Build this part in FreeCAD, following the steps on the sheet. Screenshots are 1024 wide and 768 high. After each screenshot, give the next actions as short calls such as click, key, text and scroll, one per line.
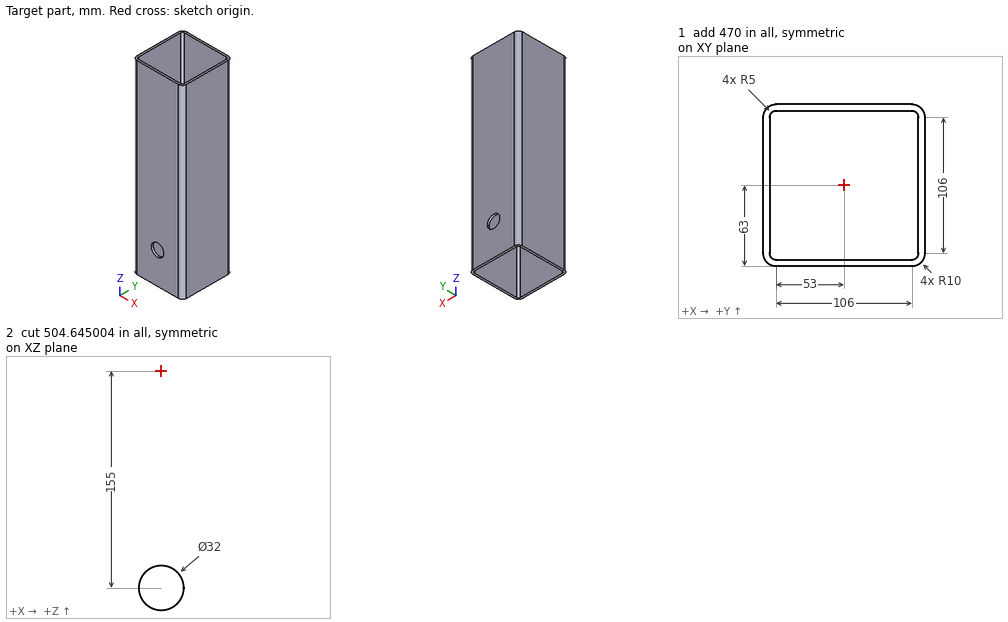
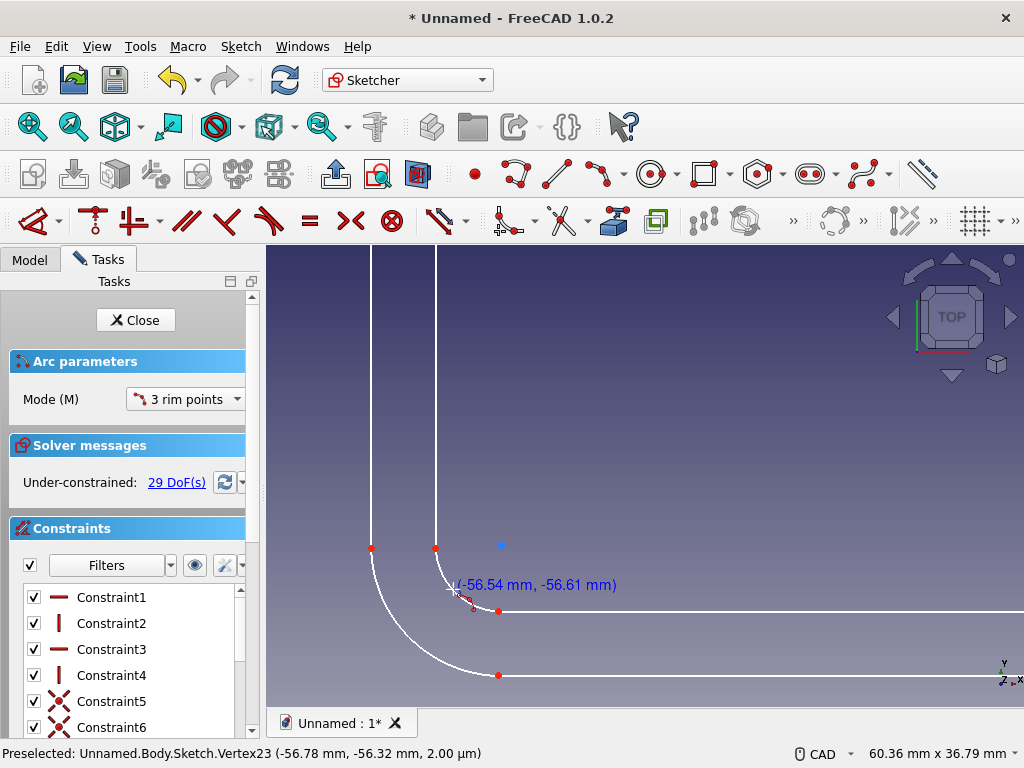
scroll(460, 594, down, 9)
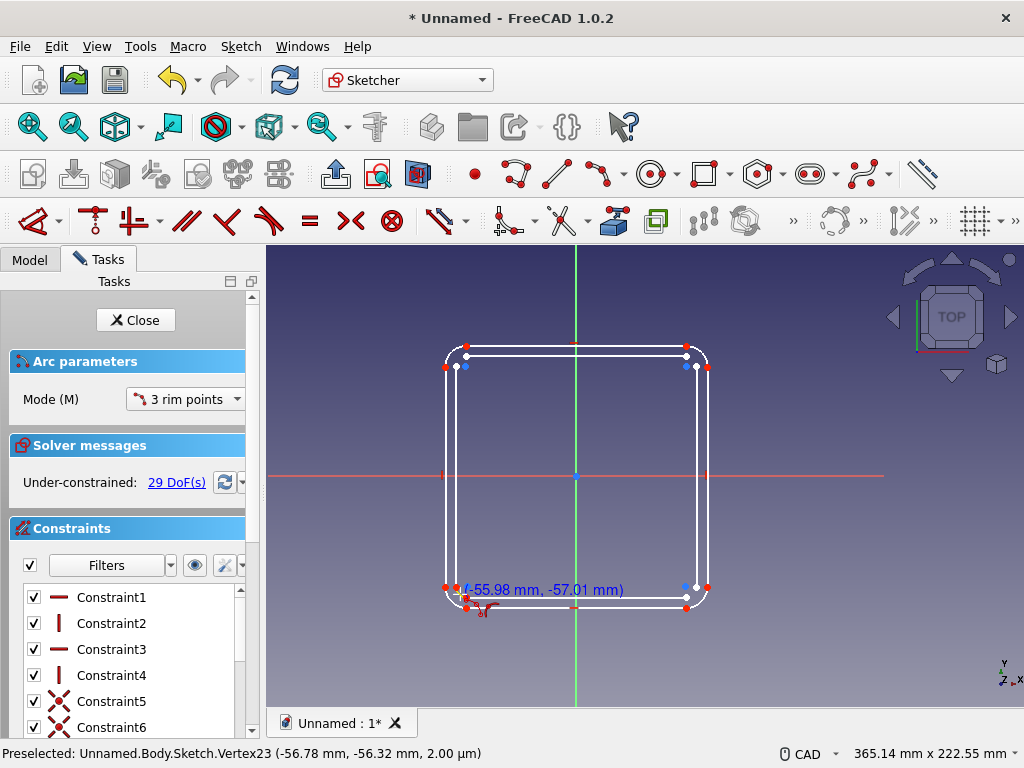
scroll(456, 366, up, 3)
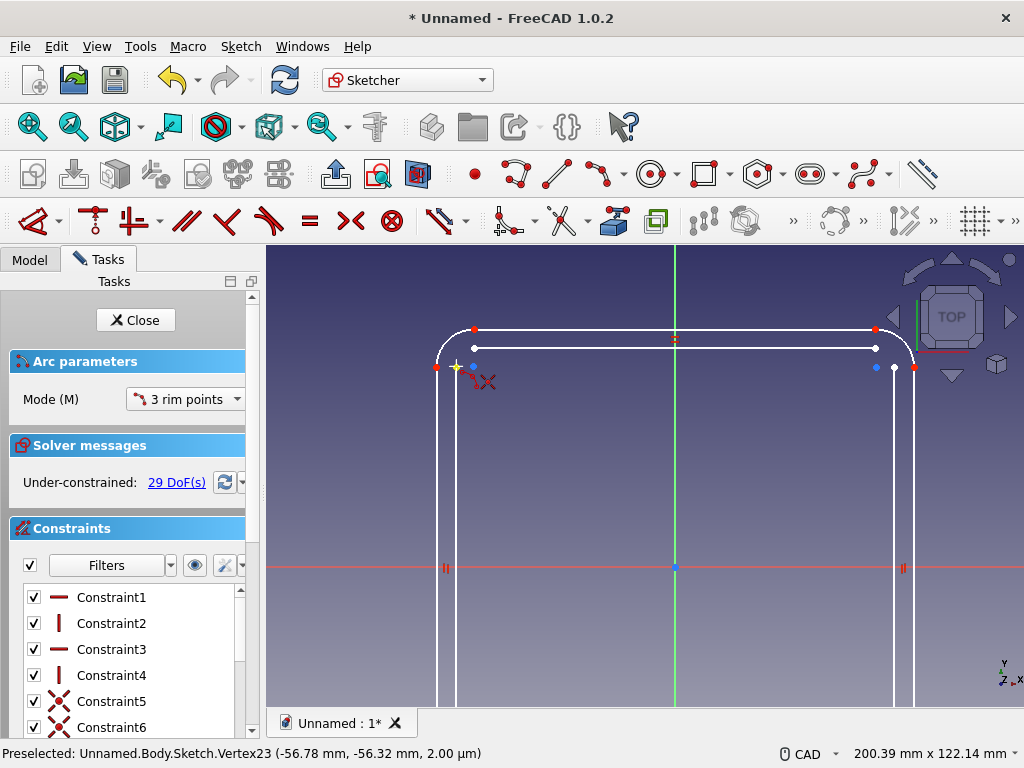
click(456, 367)
click(475, 348)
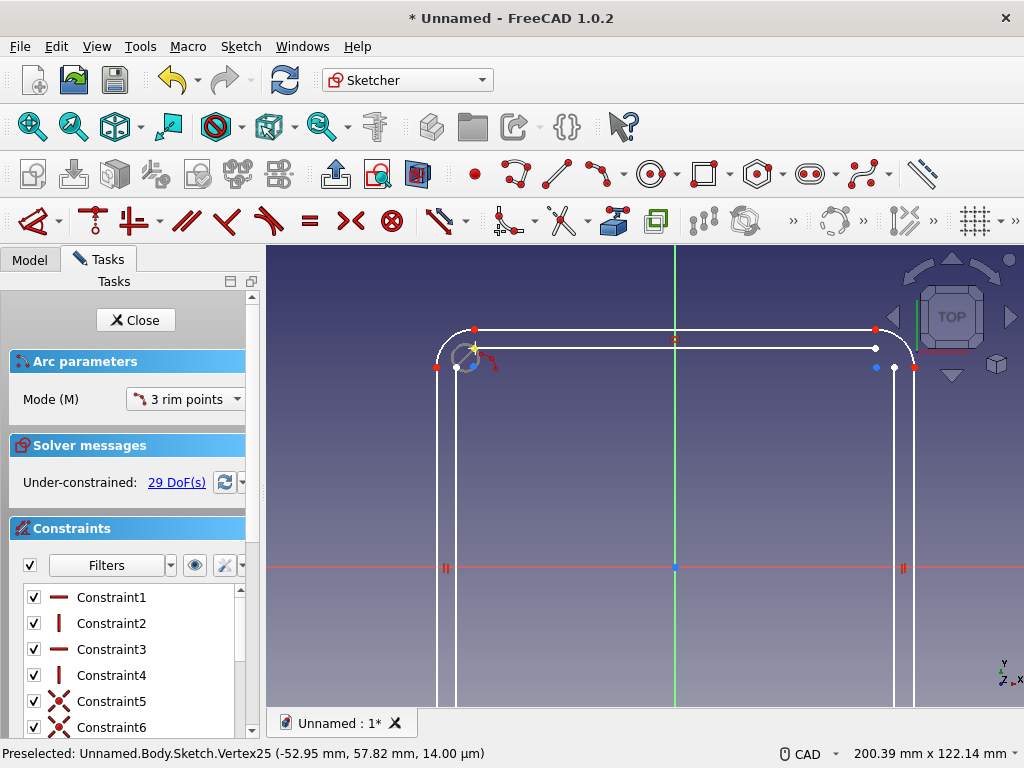
scroll(461, 353, up, 6)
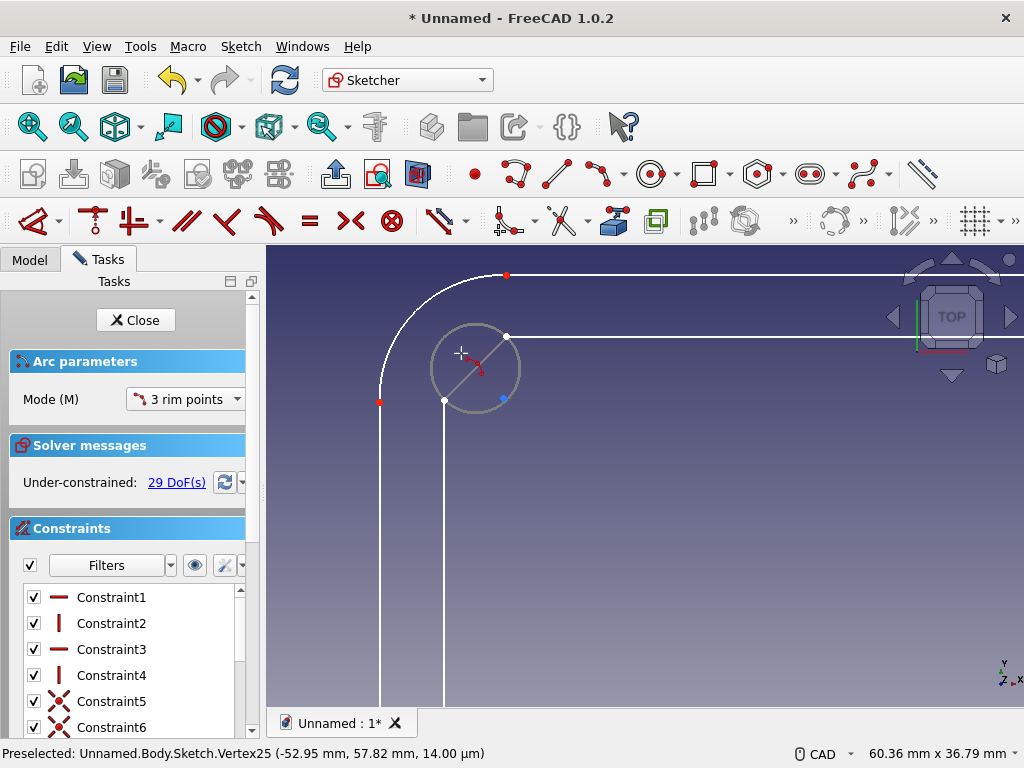
click(462, 353)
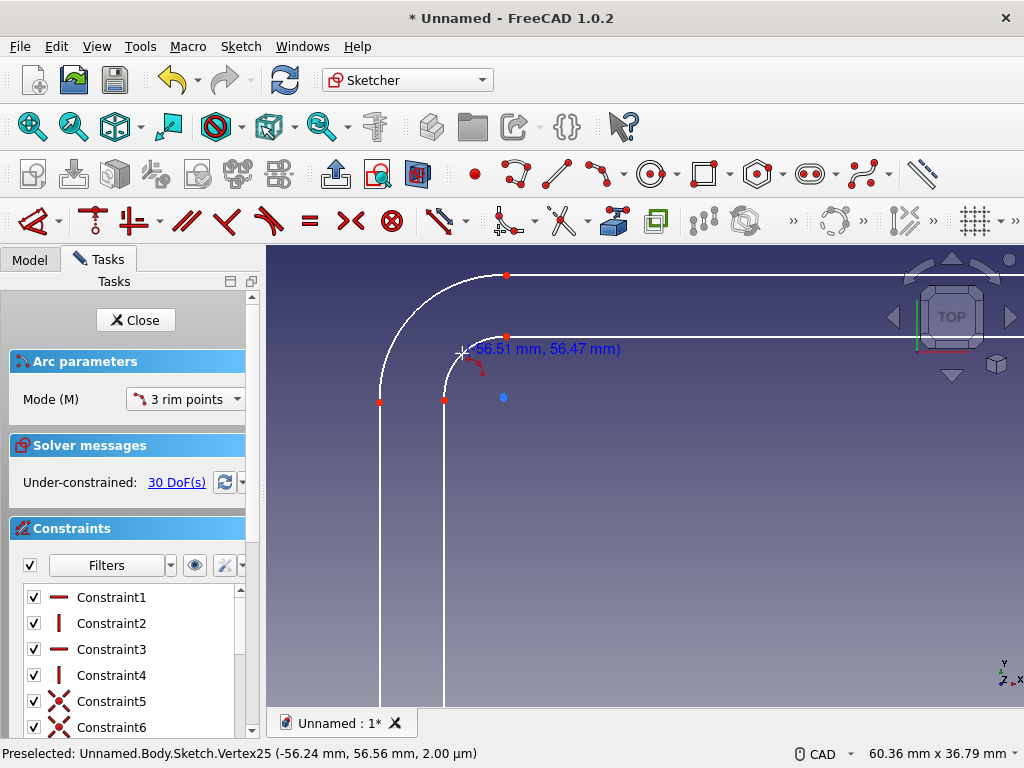
scroll(459, 360, down, 9)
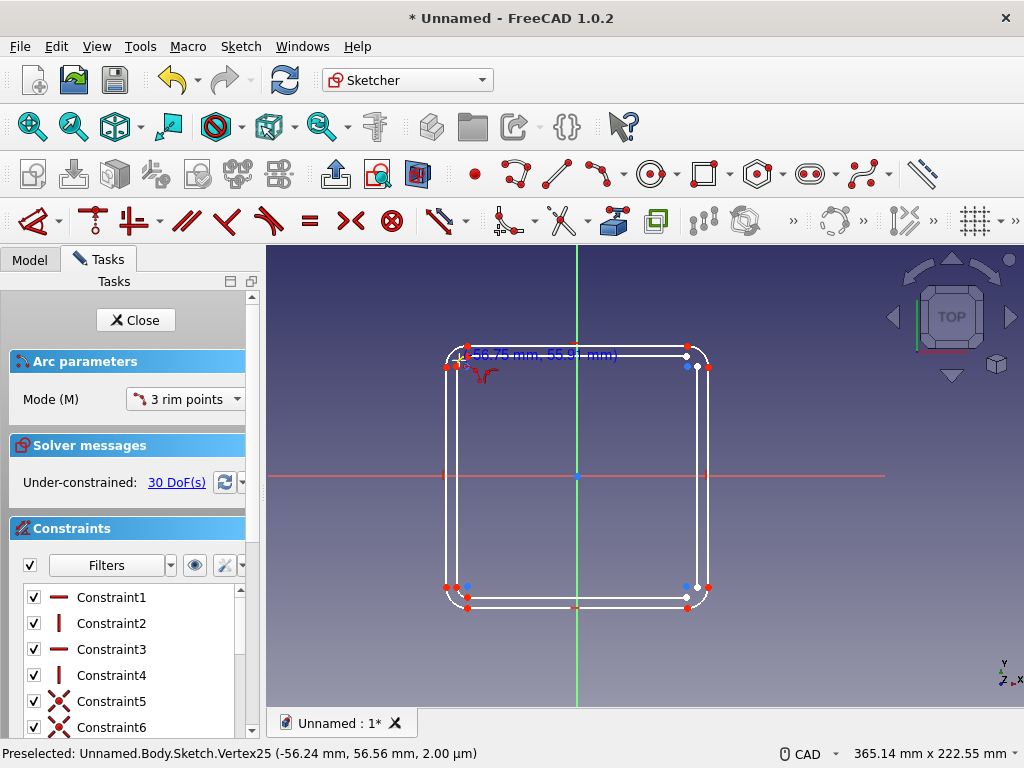
scroll(687, 356, up, 3)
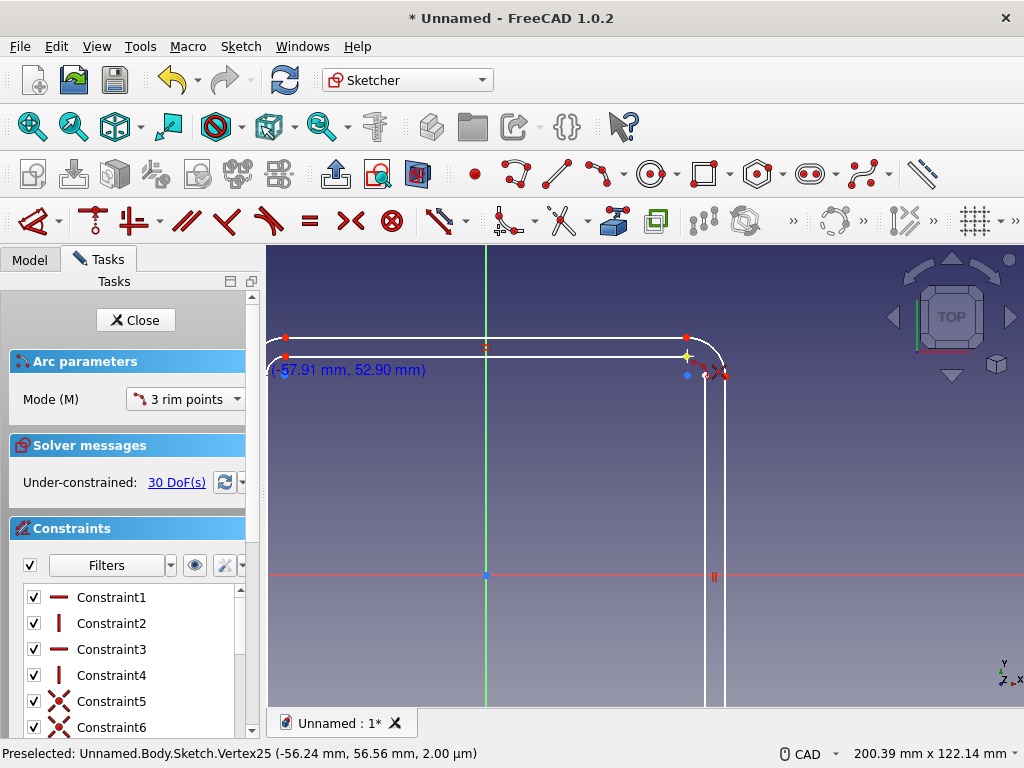
click(686, 357)
click(705, 375)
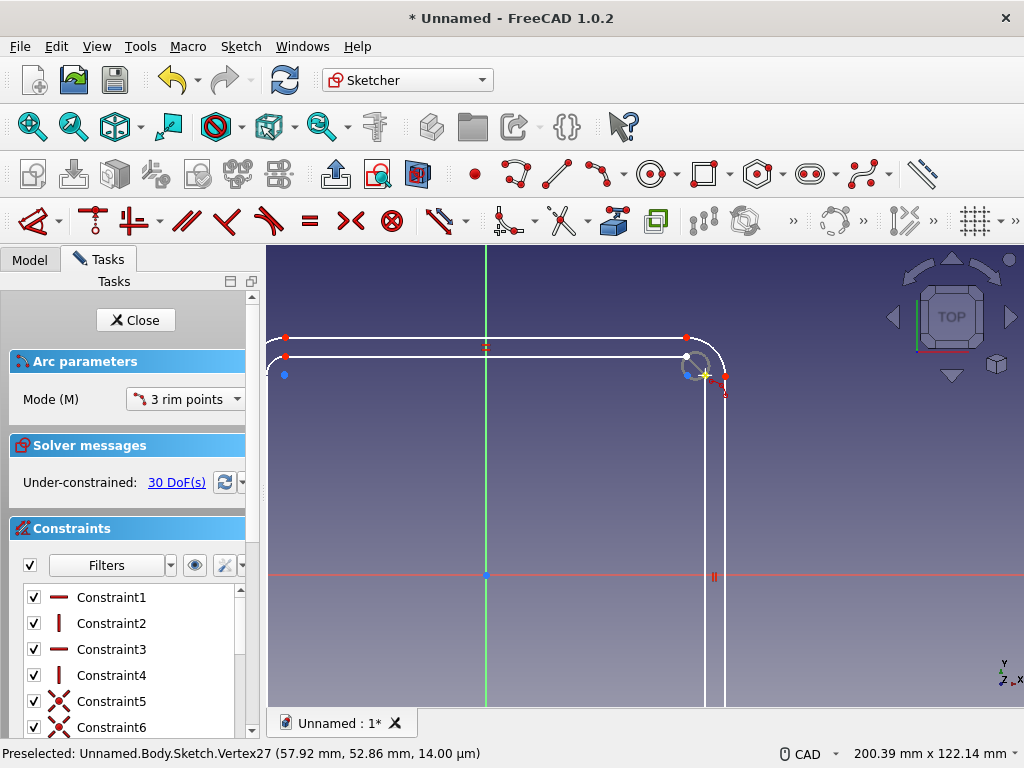
scroll(700, 361, up, 6)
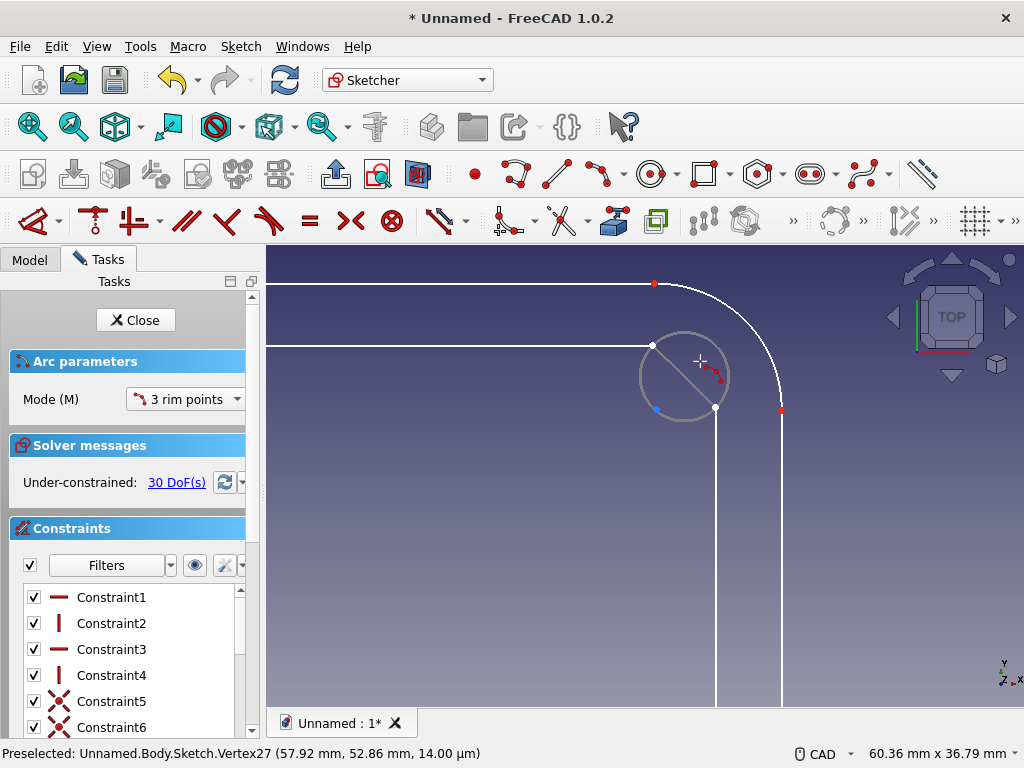
click(699, 362)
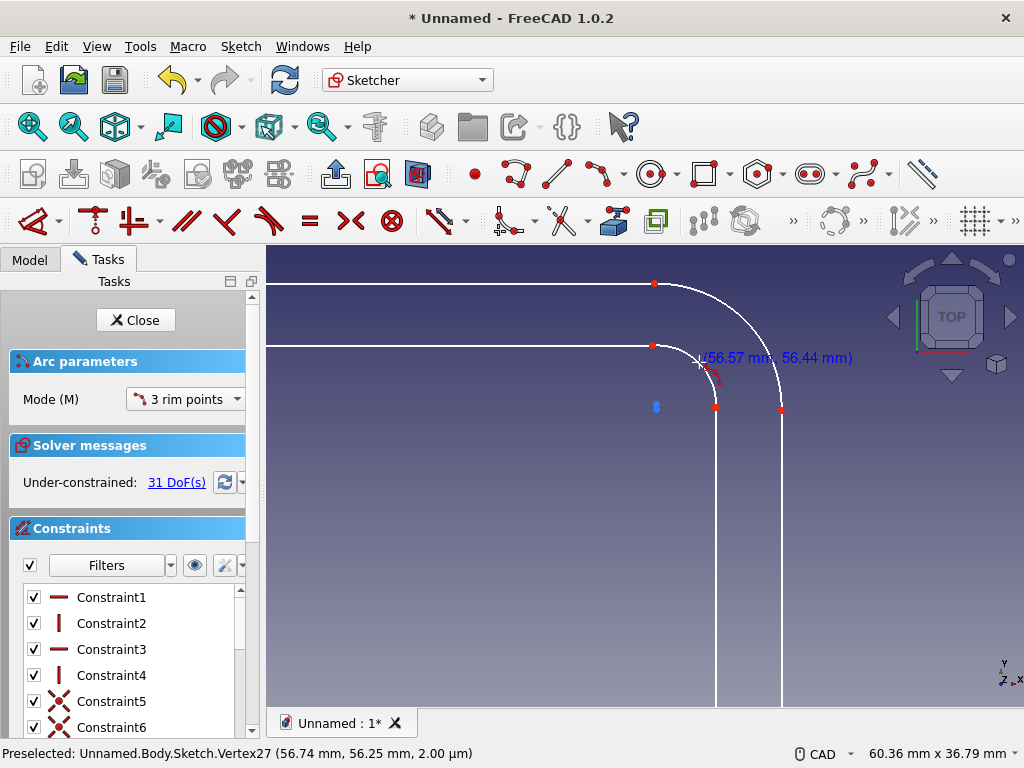
scroll(693, 358, down, 9)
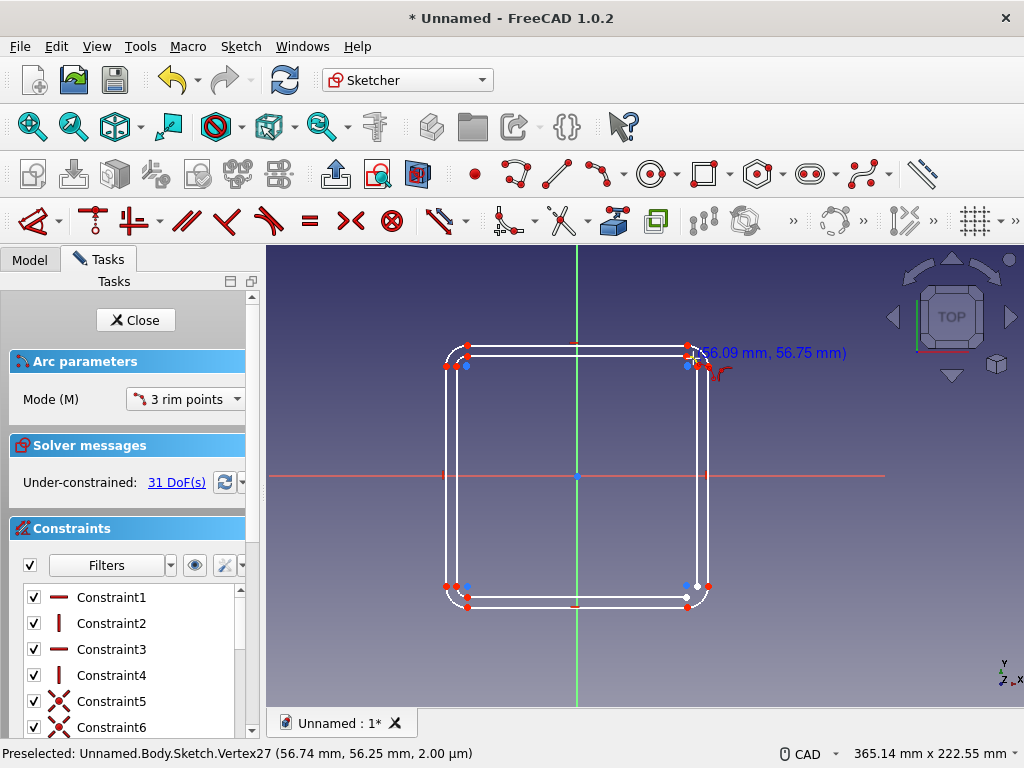
scroll(697, 586, up, 3)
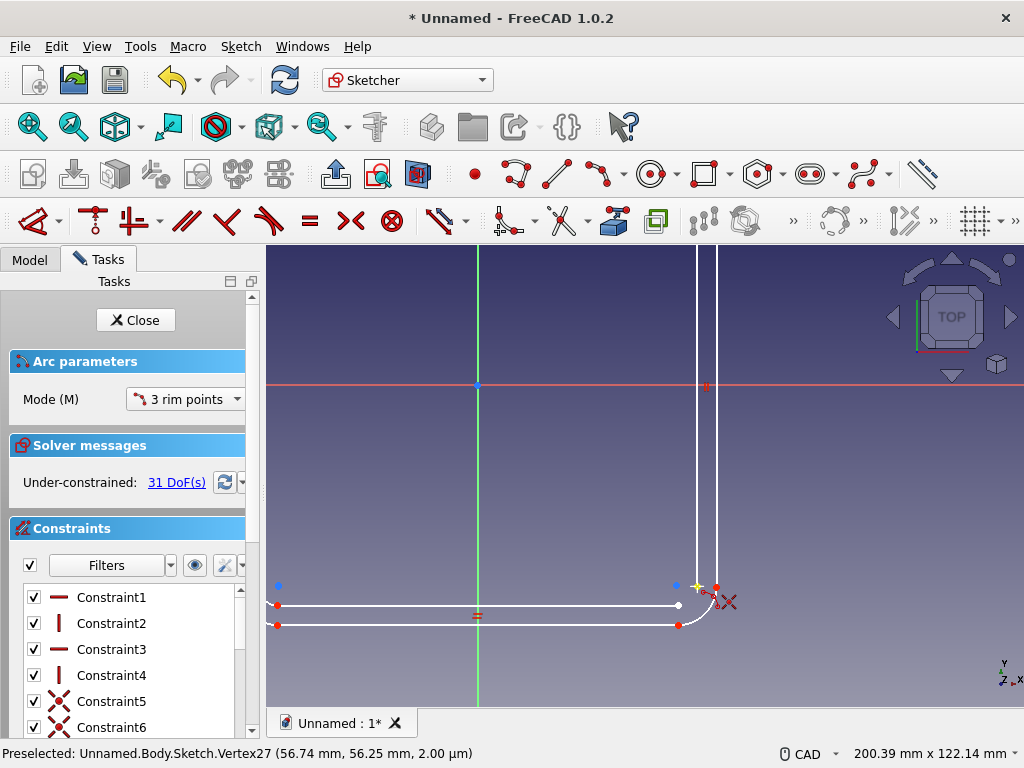
click(697, 587)
click(678, 606)